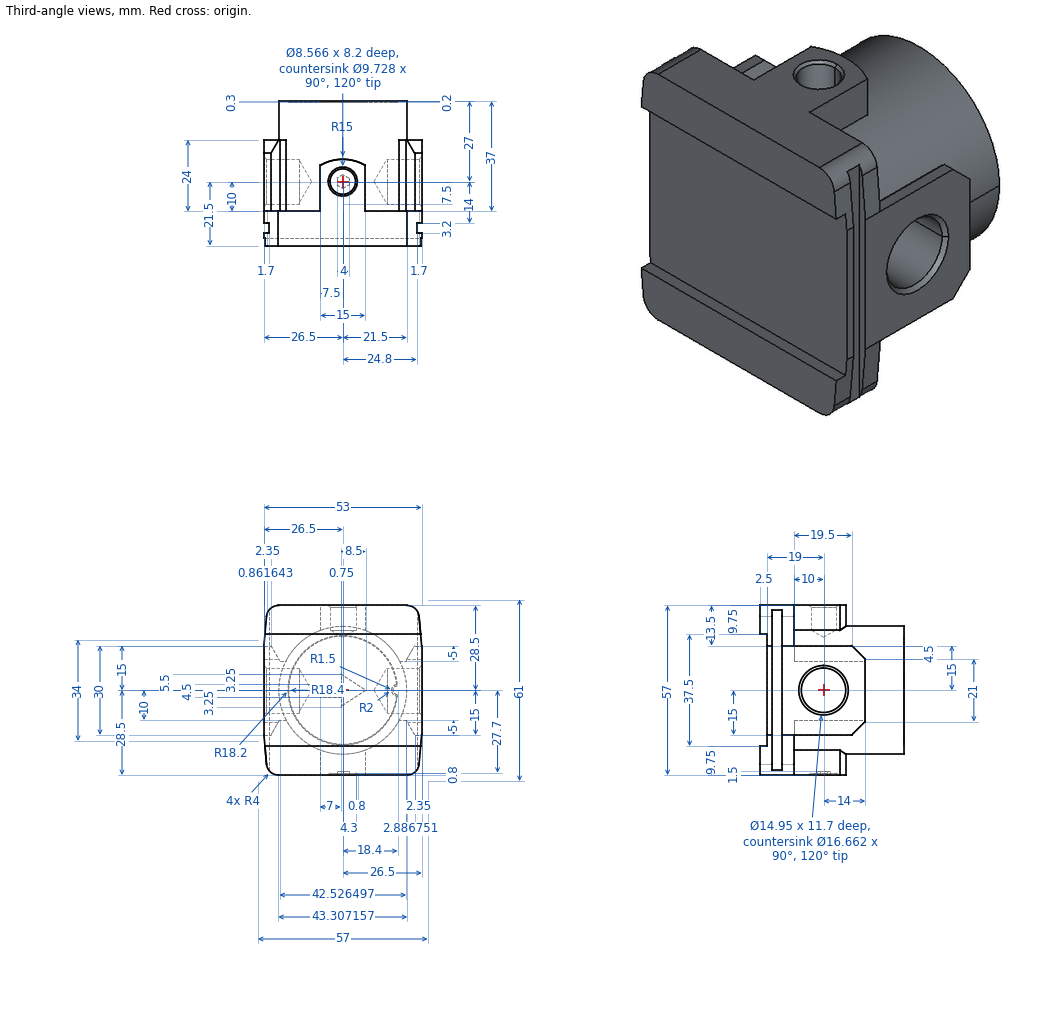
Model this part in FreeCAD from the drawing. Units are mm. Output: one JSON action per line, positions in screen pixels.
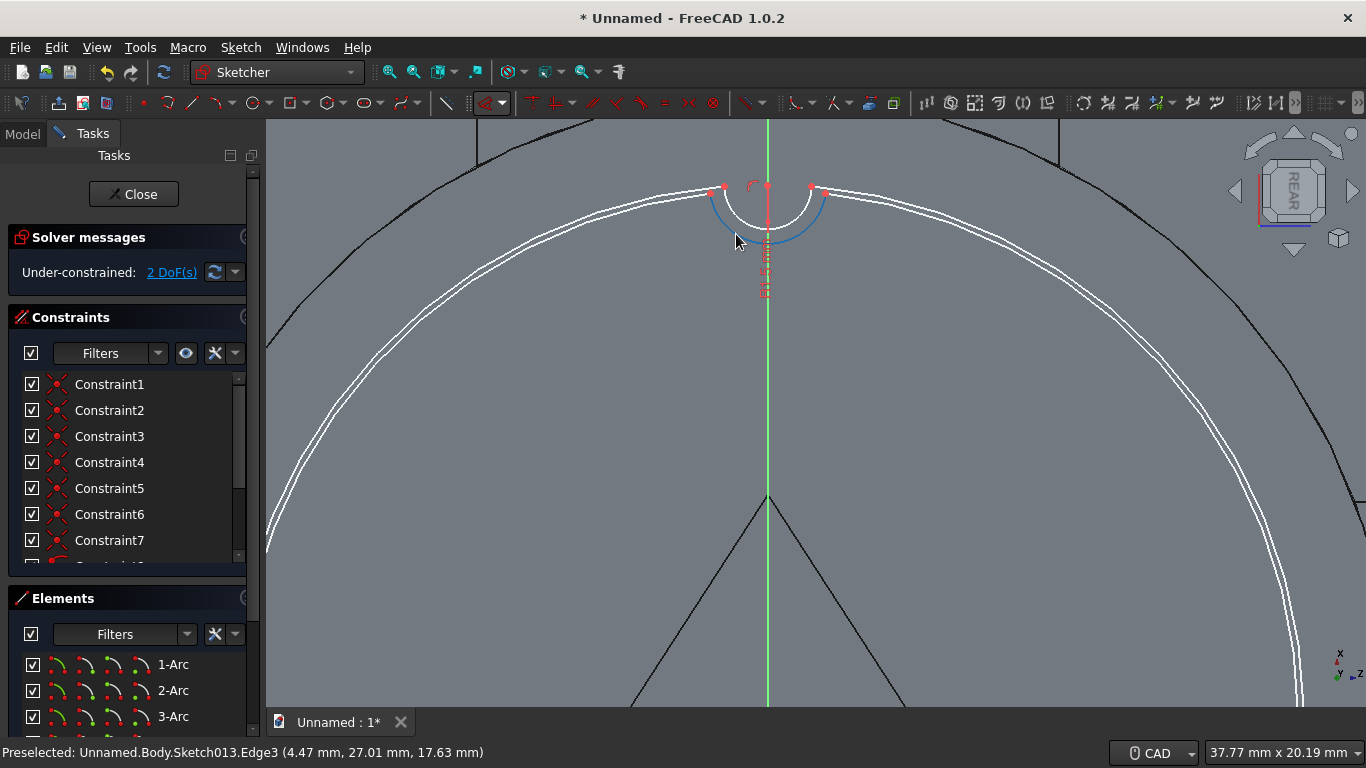
{"action": "left_click", "coordinate": [736, 235]}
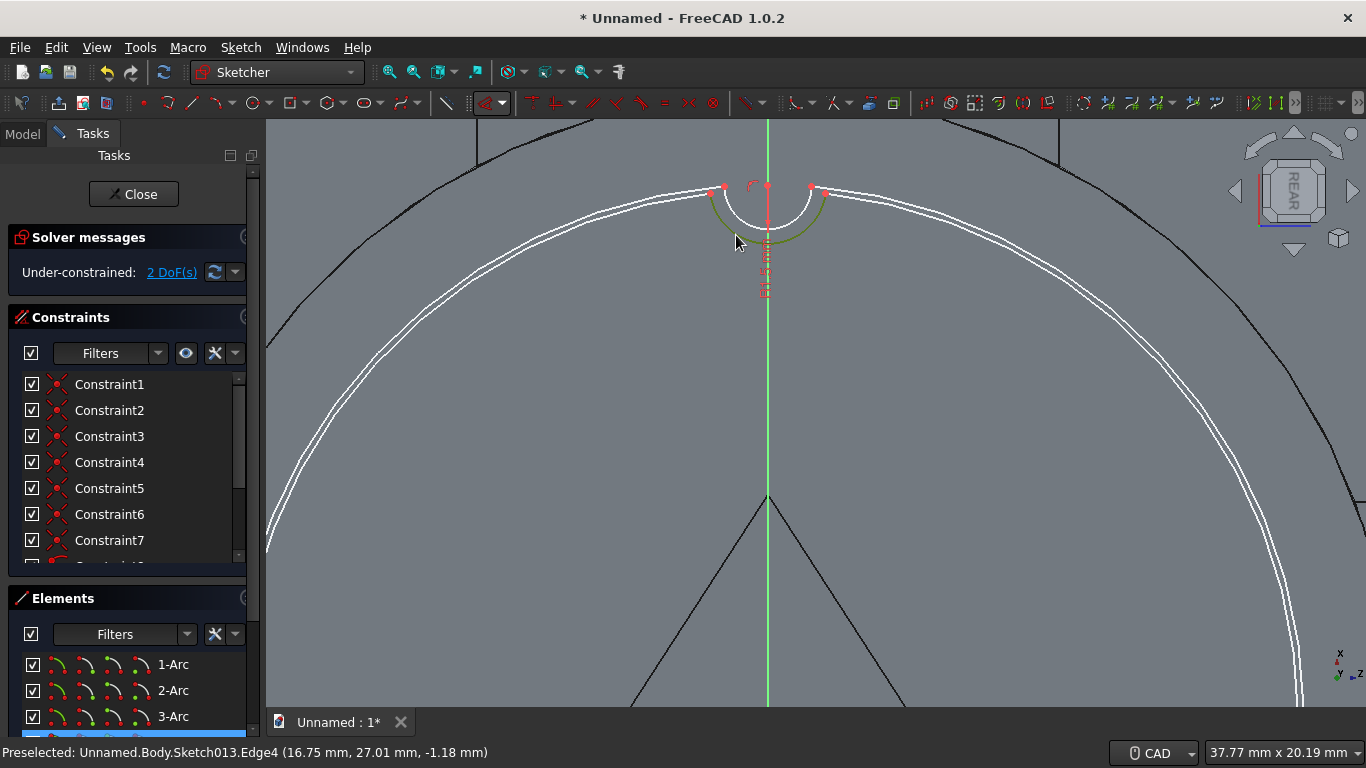
{"action": "key", "text": "k r"}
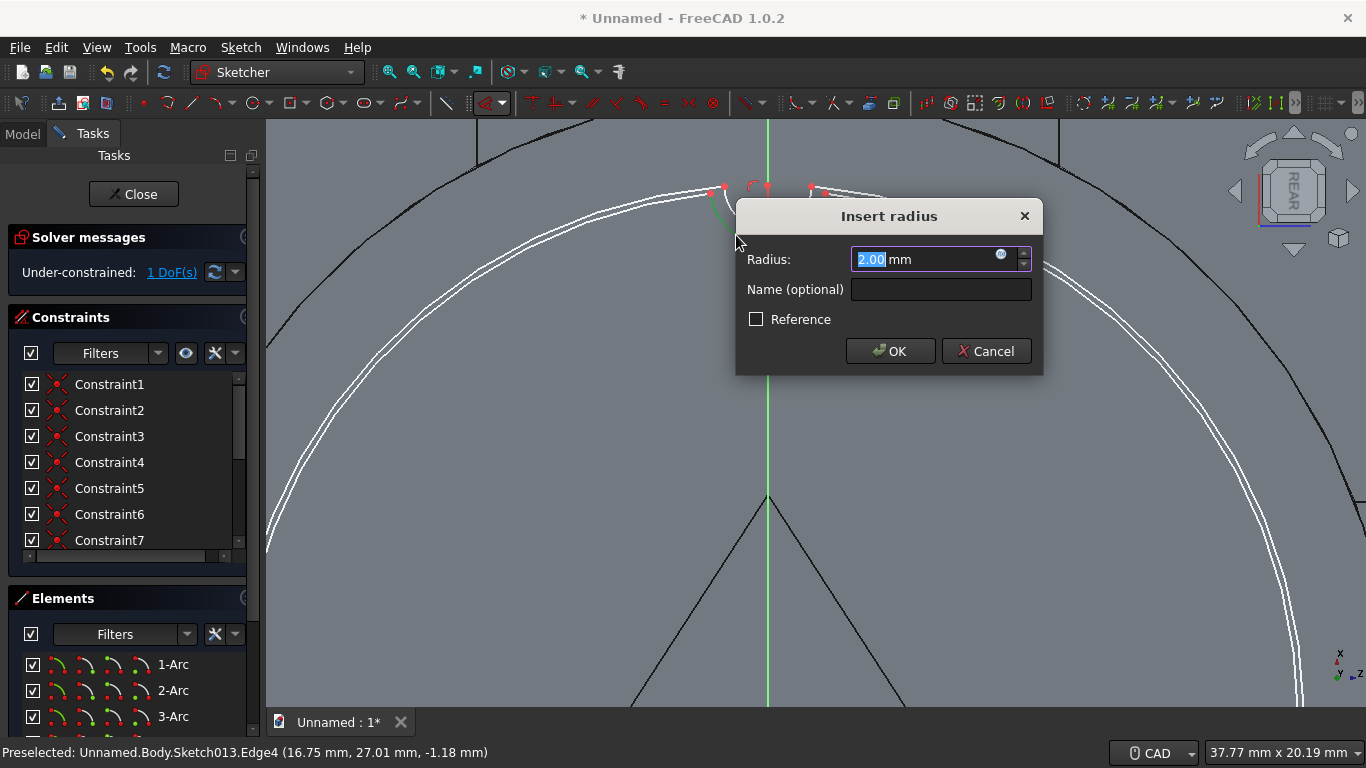
{"action": "type", "text": "2"}
{"action": "key", "text": "Return"}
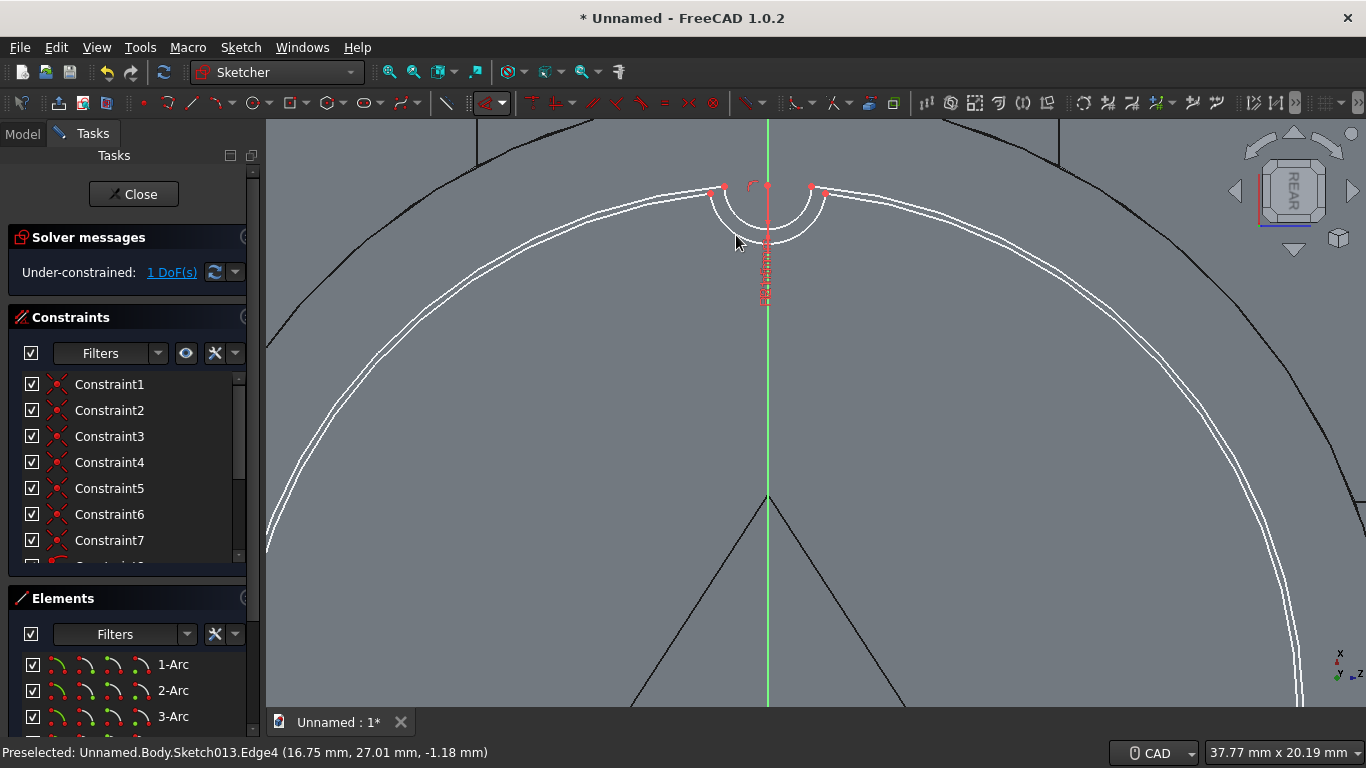
{"action": "left_click", "coordinate": [768, 186]}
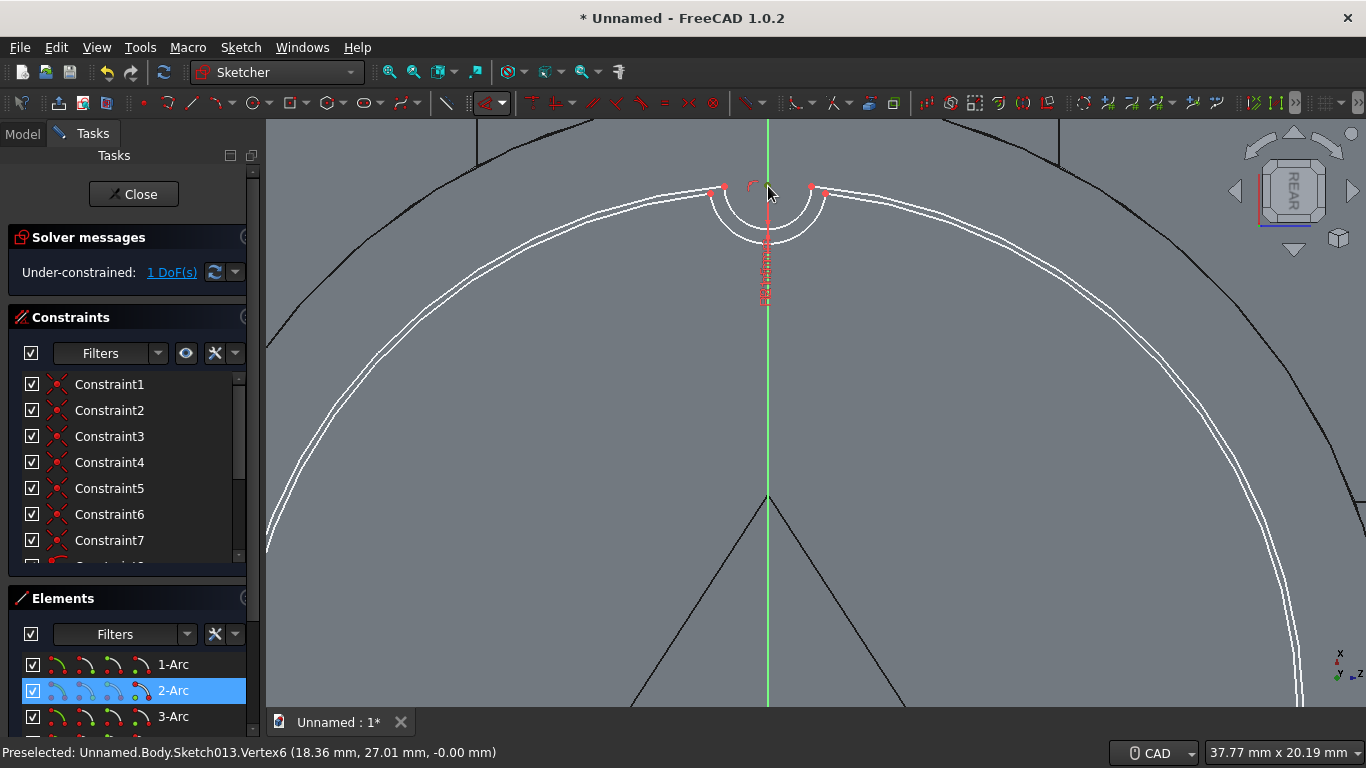
{"action": "left_click", "coordinate": [504, 104]}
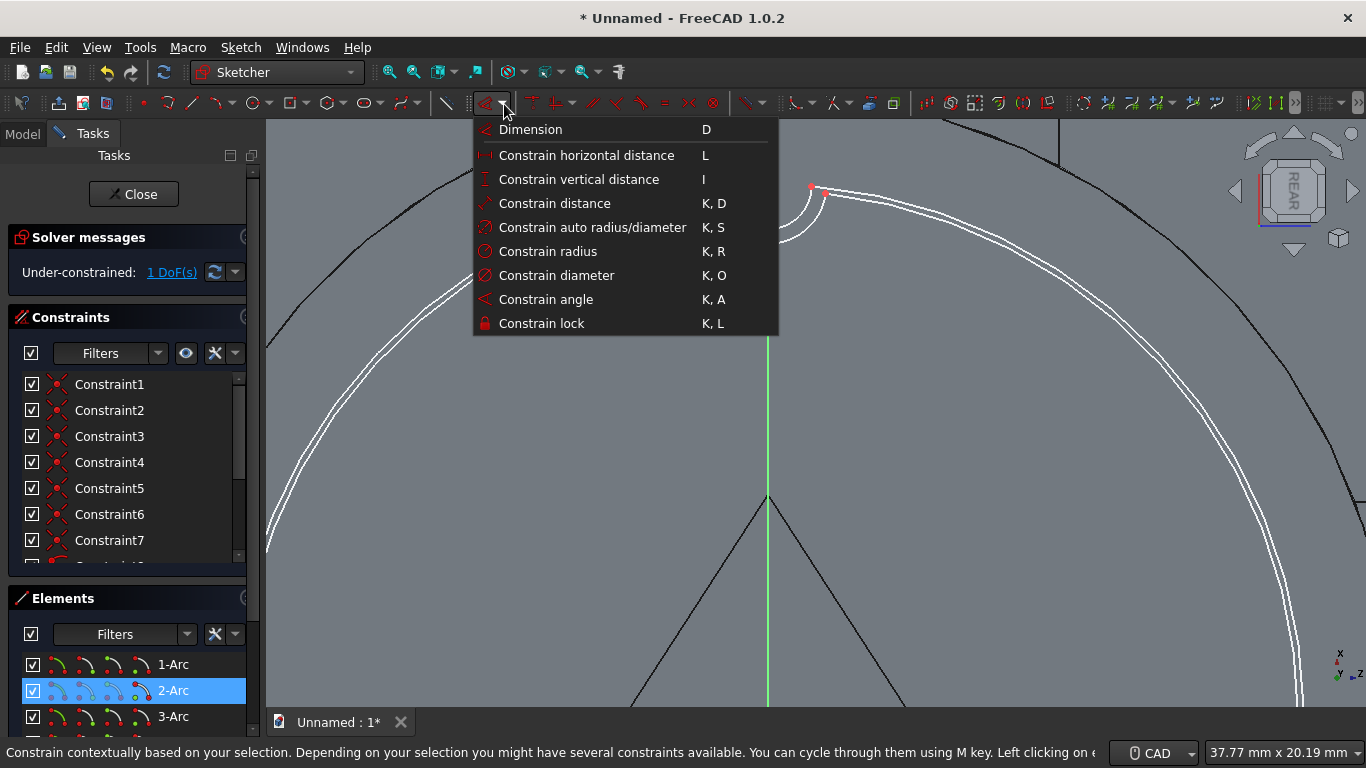
{"action": "left_click", "coordinate": [626, 179]}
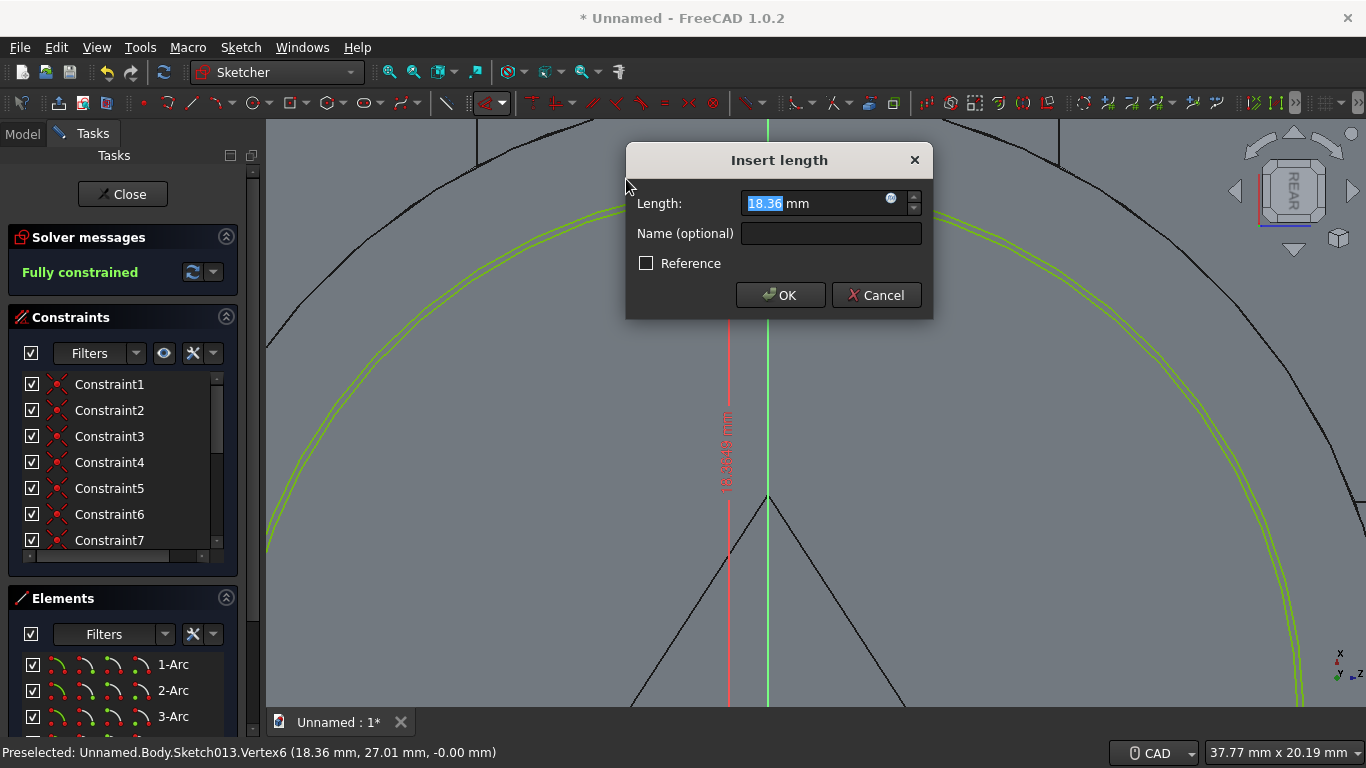
{"action": "type", "text": "18.4"}
{"action": "key", "text": "Return"}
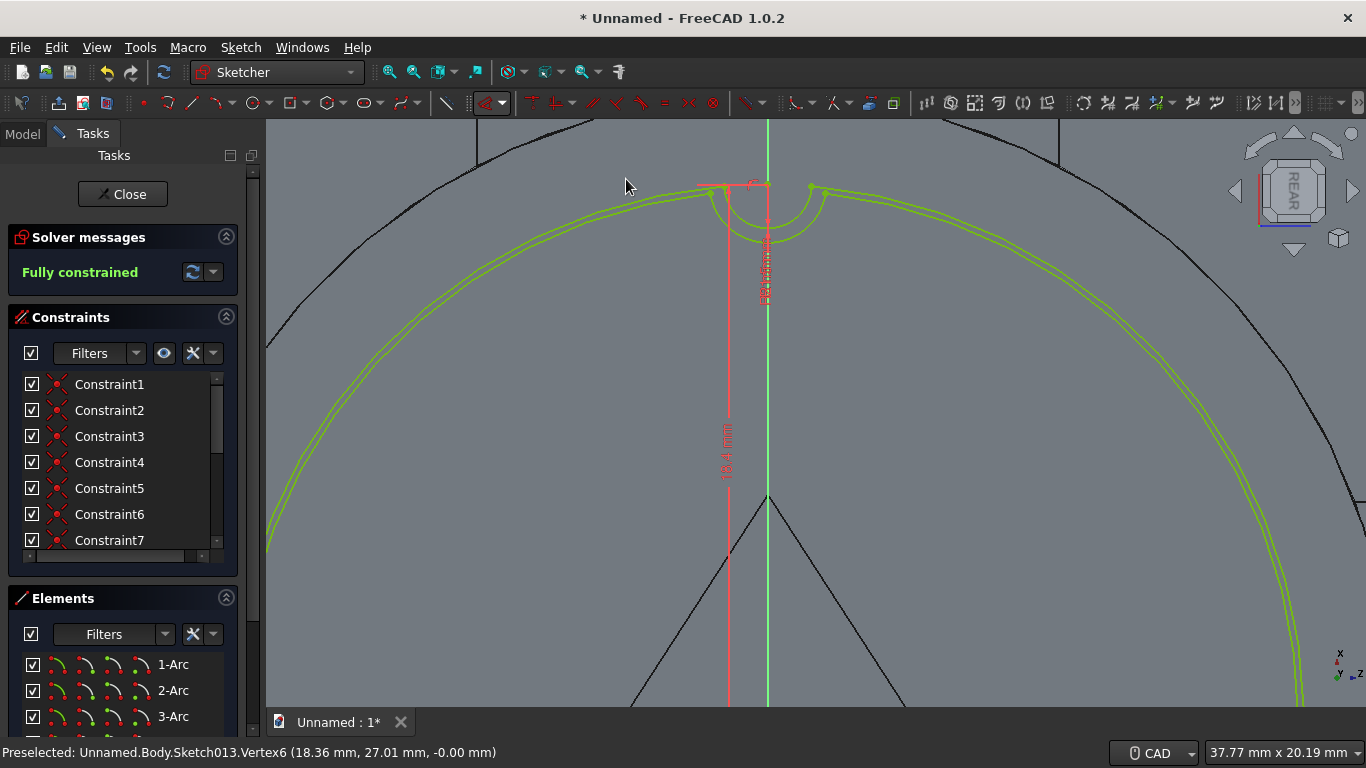
{"action": "left_click", "coordinate": [123, 194]}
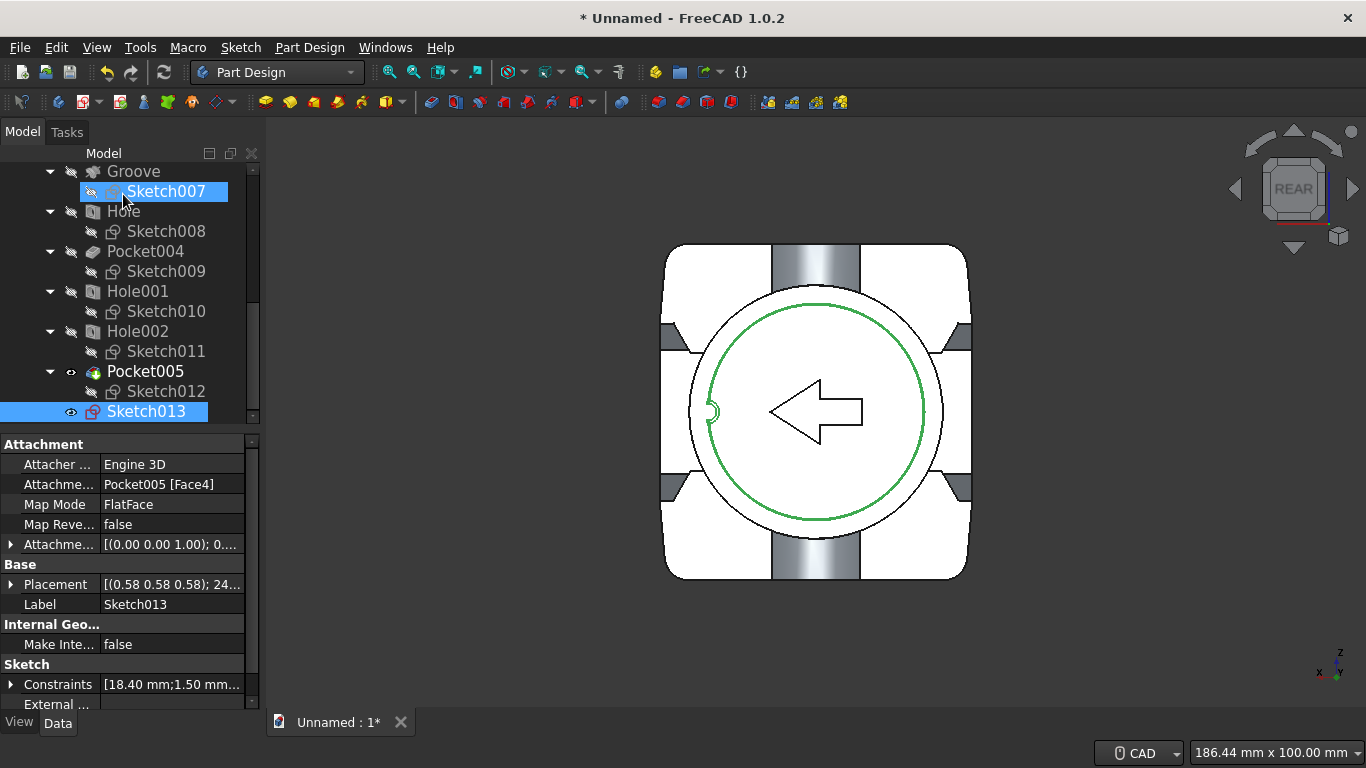
{"action": "left_click", "coordinate": [432, 102]}